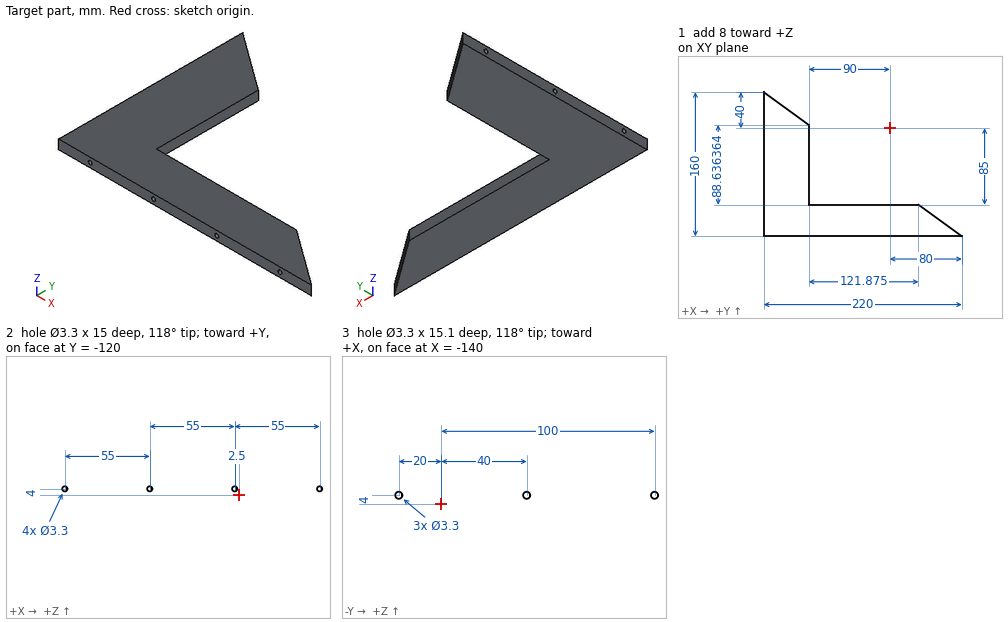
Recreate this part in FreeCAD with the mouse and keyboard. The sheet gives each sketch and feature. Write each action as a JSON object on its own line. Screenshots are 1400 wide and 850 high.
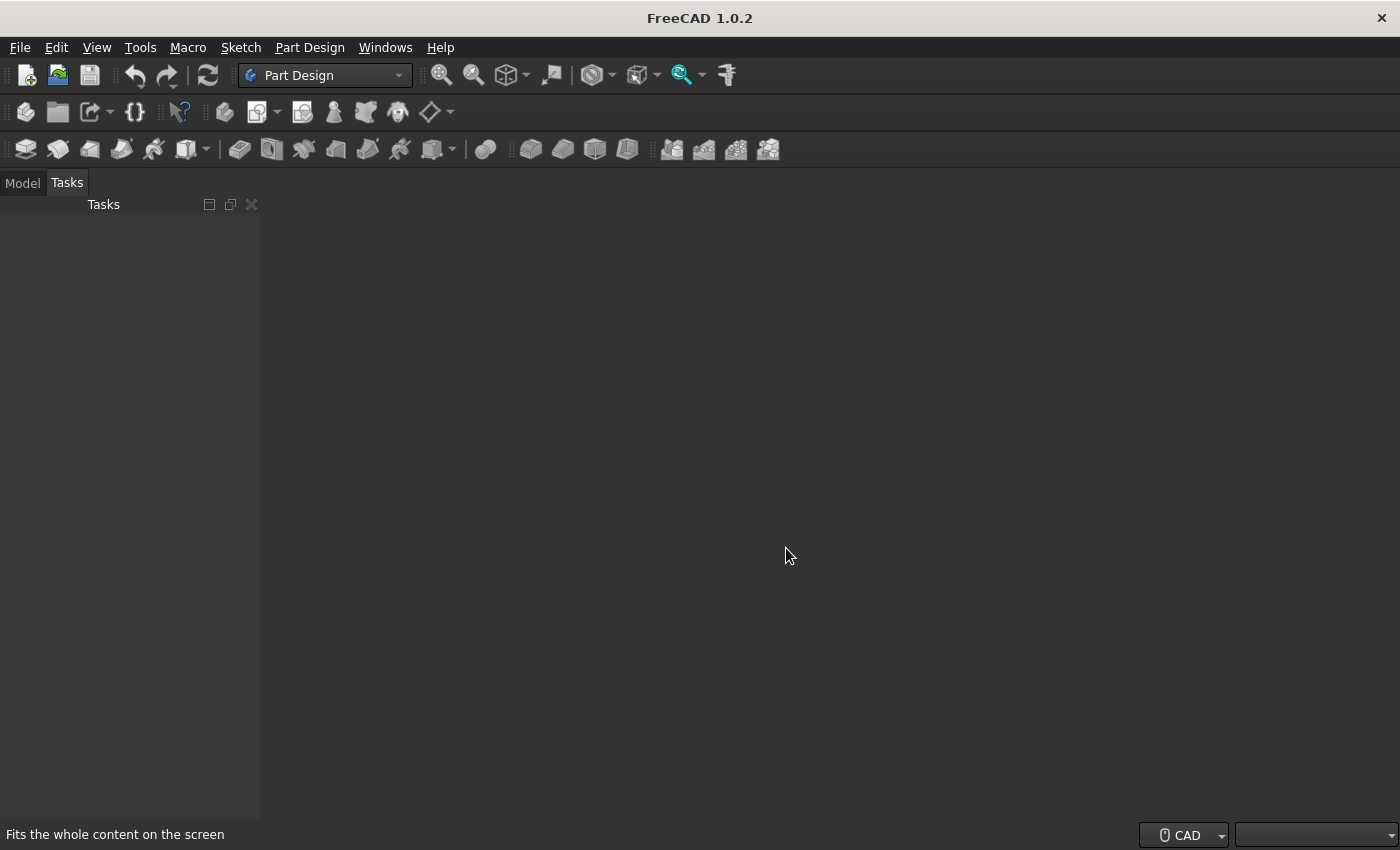
{"action": "key", "text": "ctrl+n"}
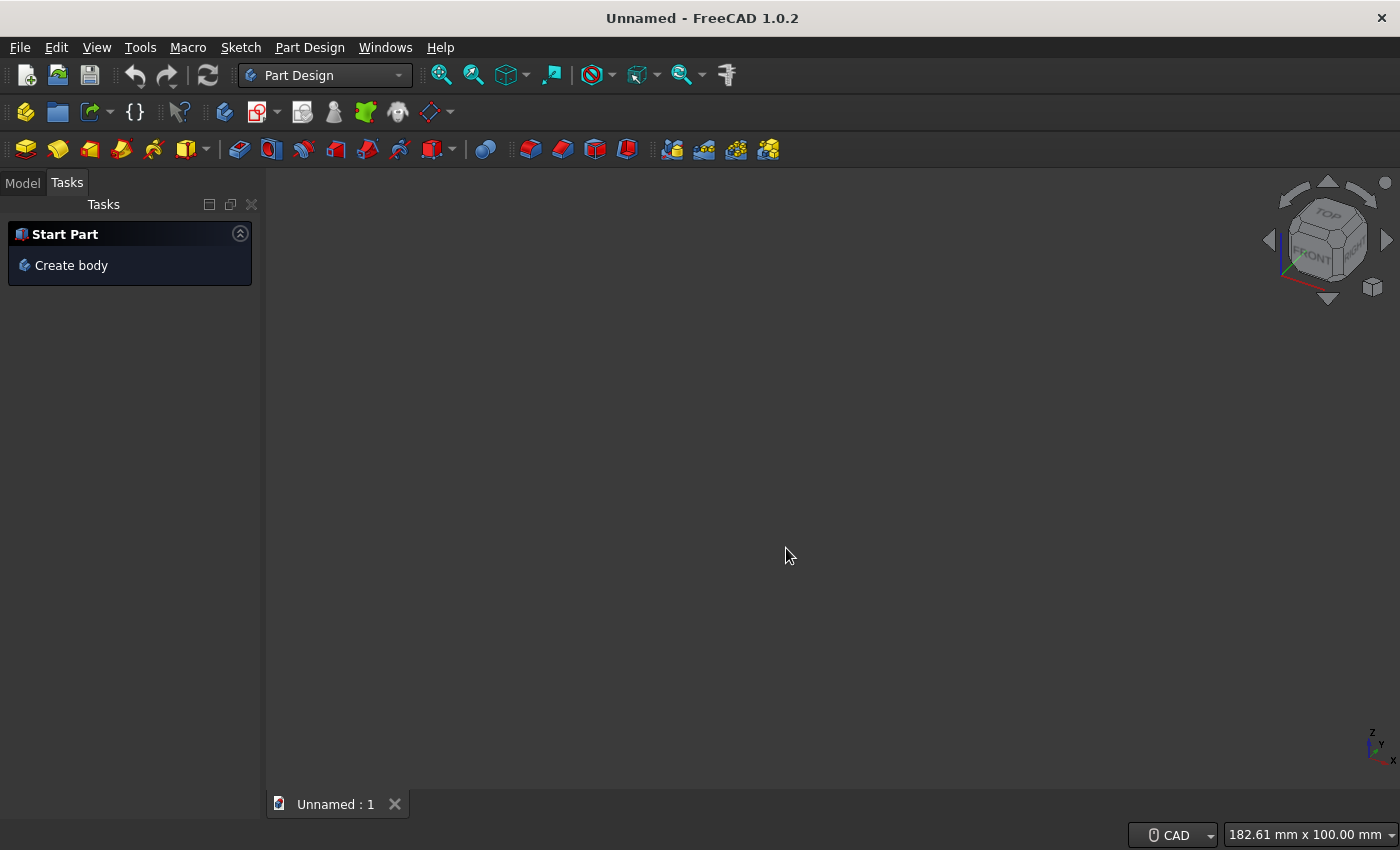
{"action": "left_click", "coordinate": [258, 112]}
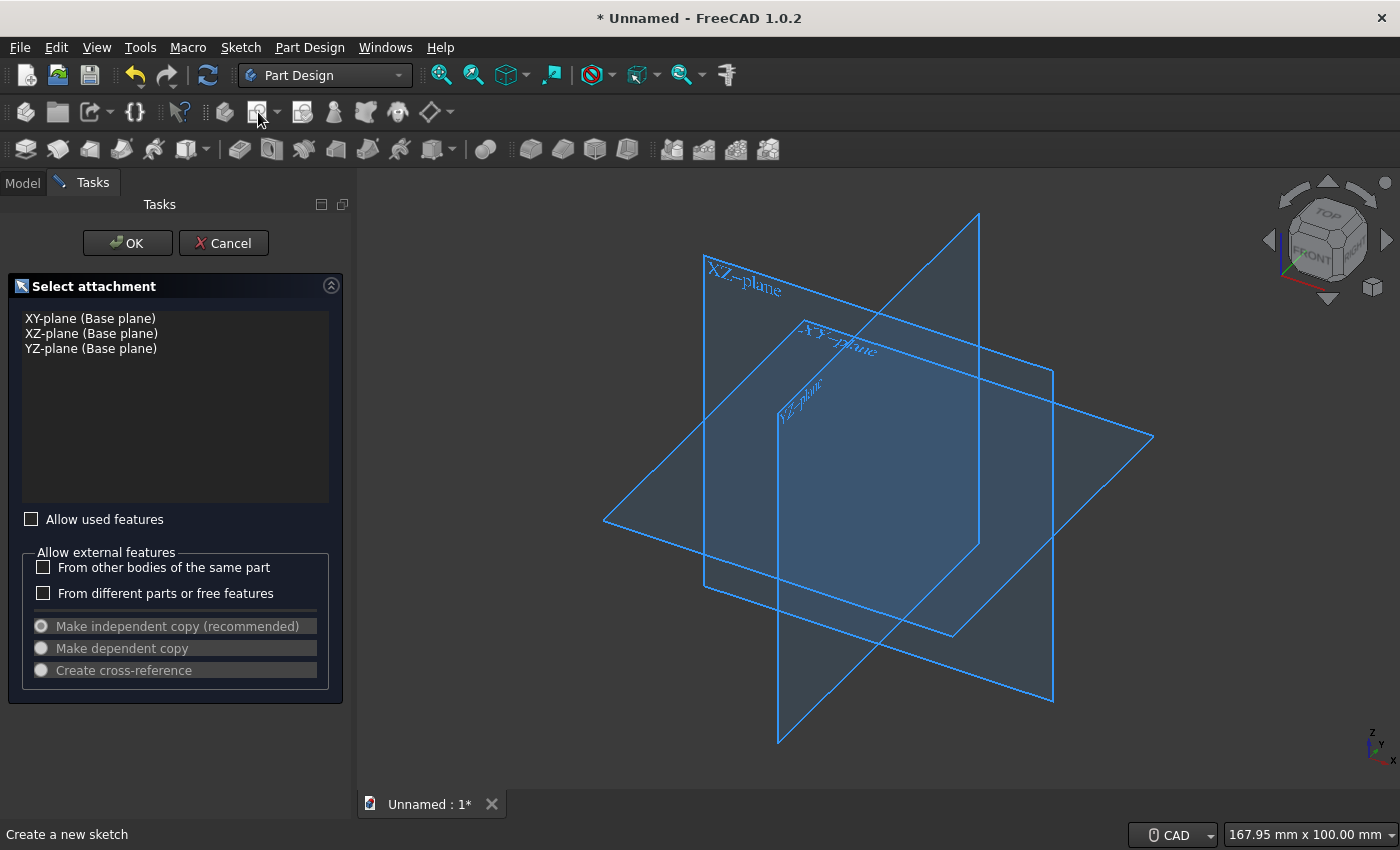
{"action": "left_click", "coordinate": [82, 318]}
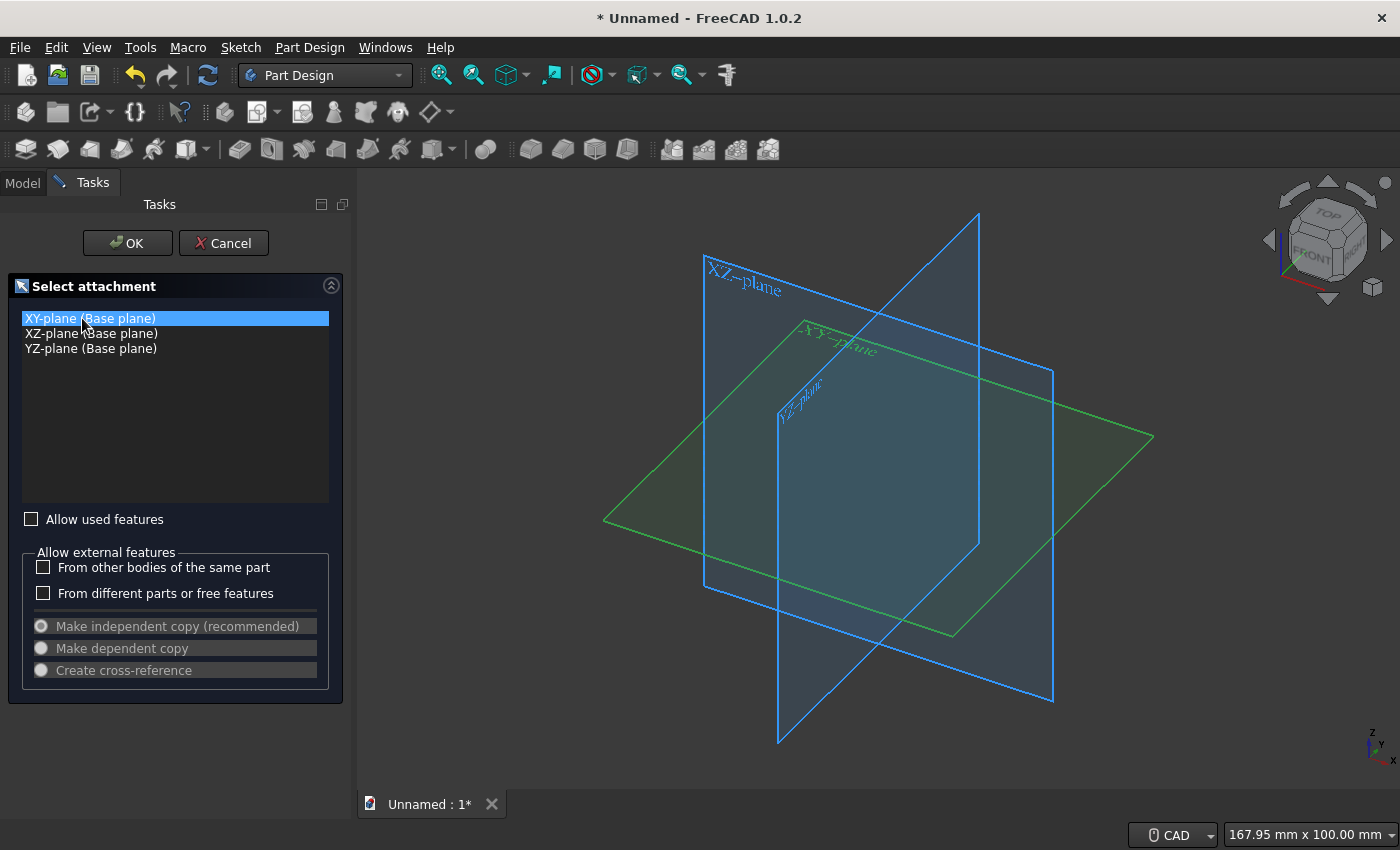
{"action": "left_click", "coordinate": [128, 243]}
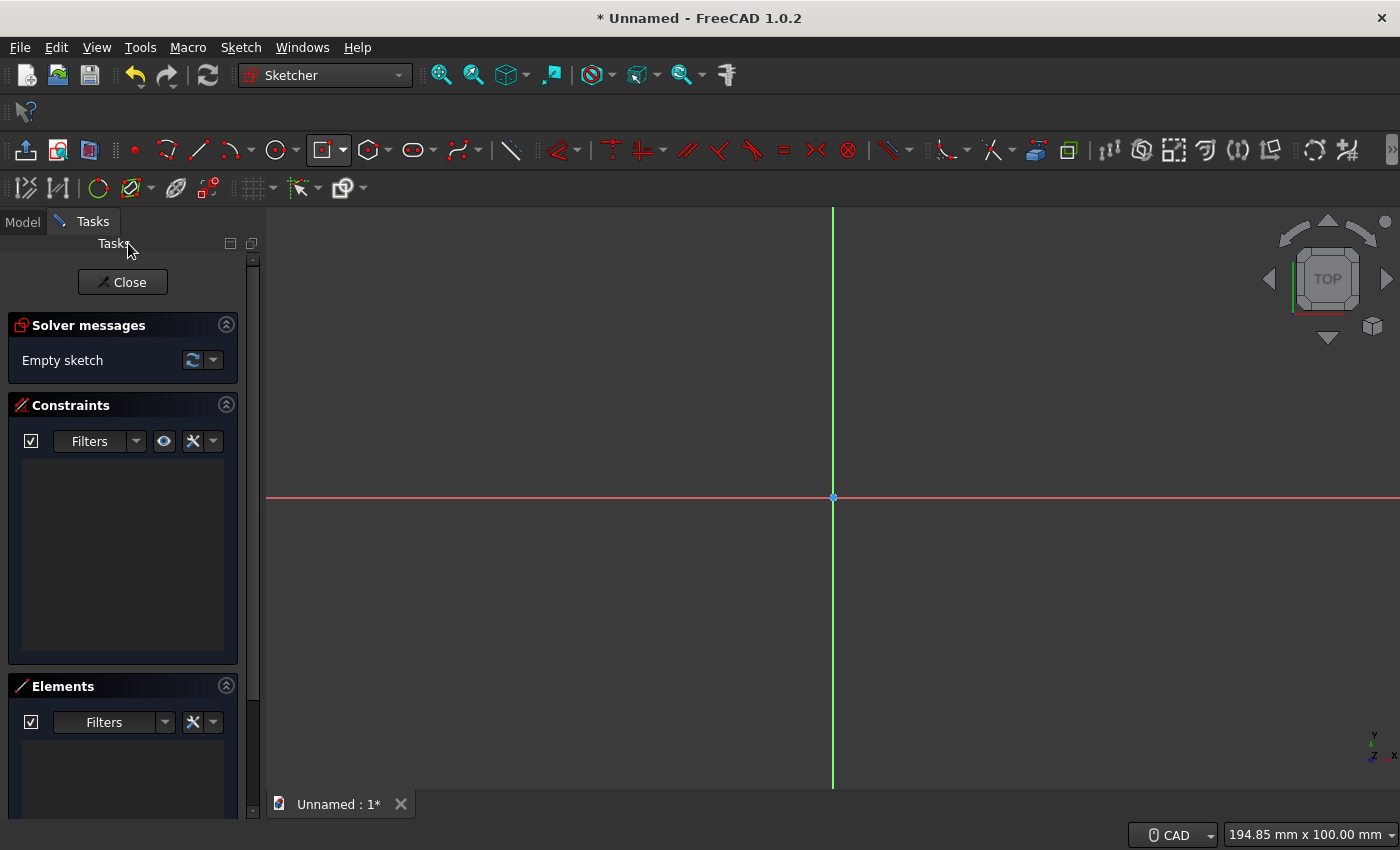
{"action": "scroll", "coordinate": [826, 363], "scroll_direction": "down", "scroll_amount": 5}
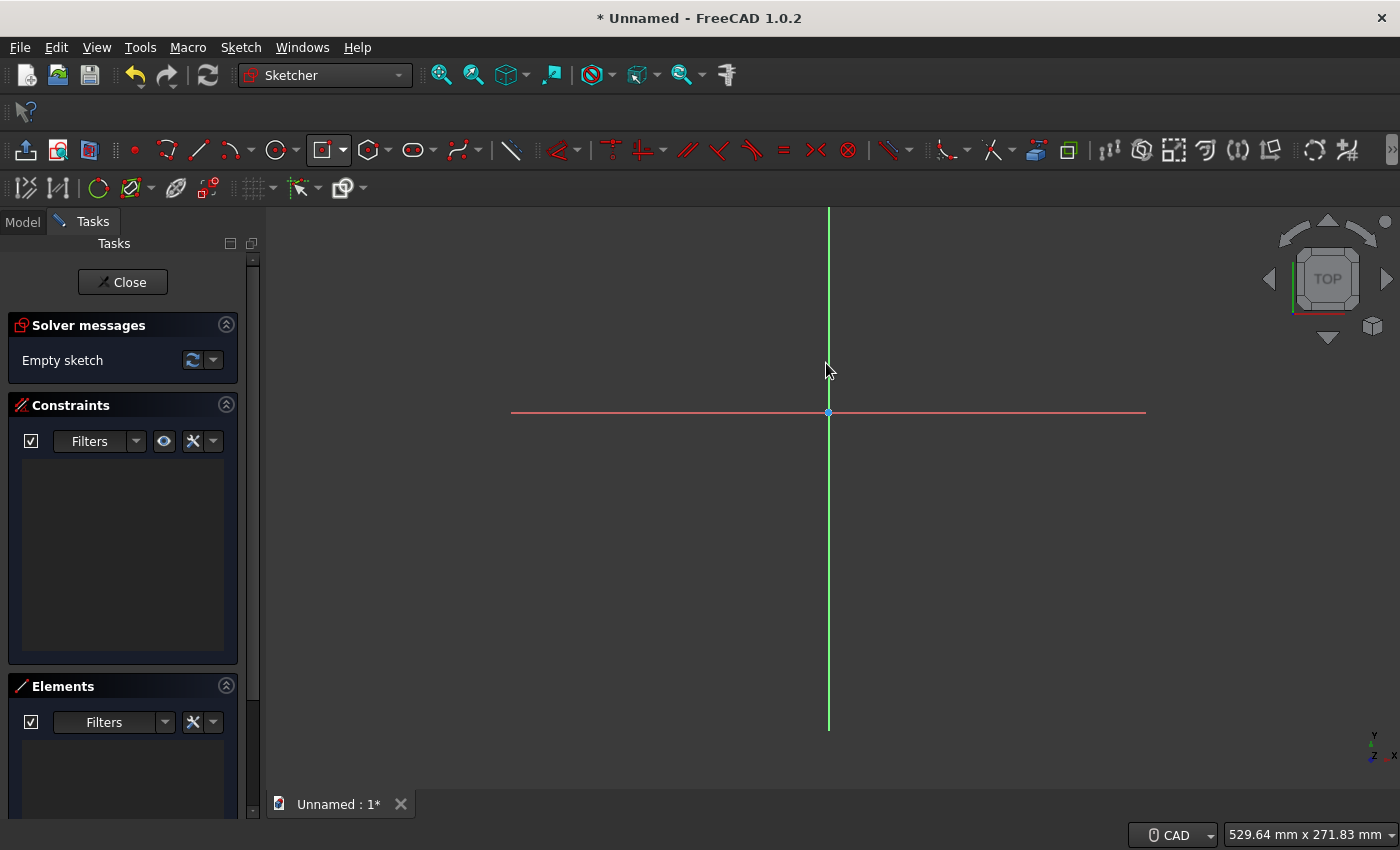
{"action": "key", "text": "g m"}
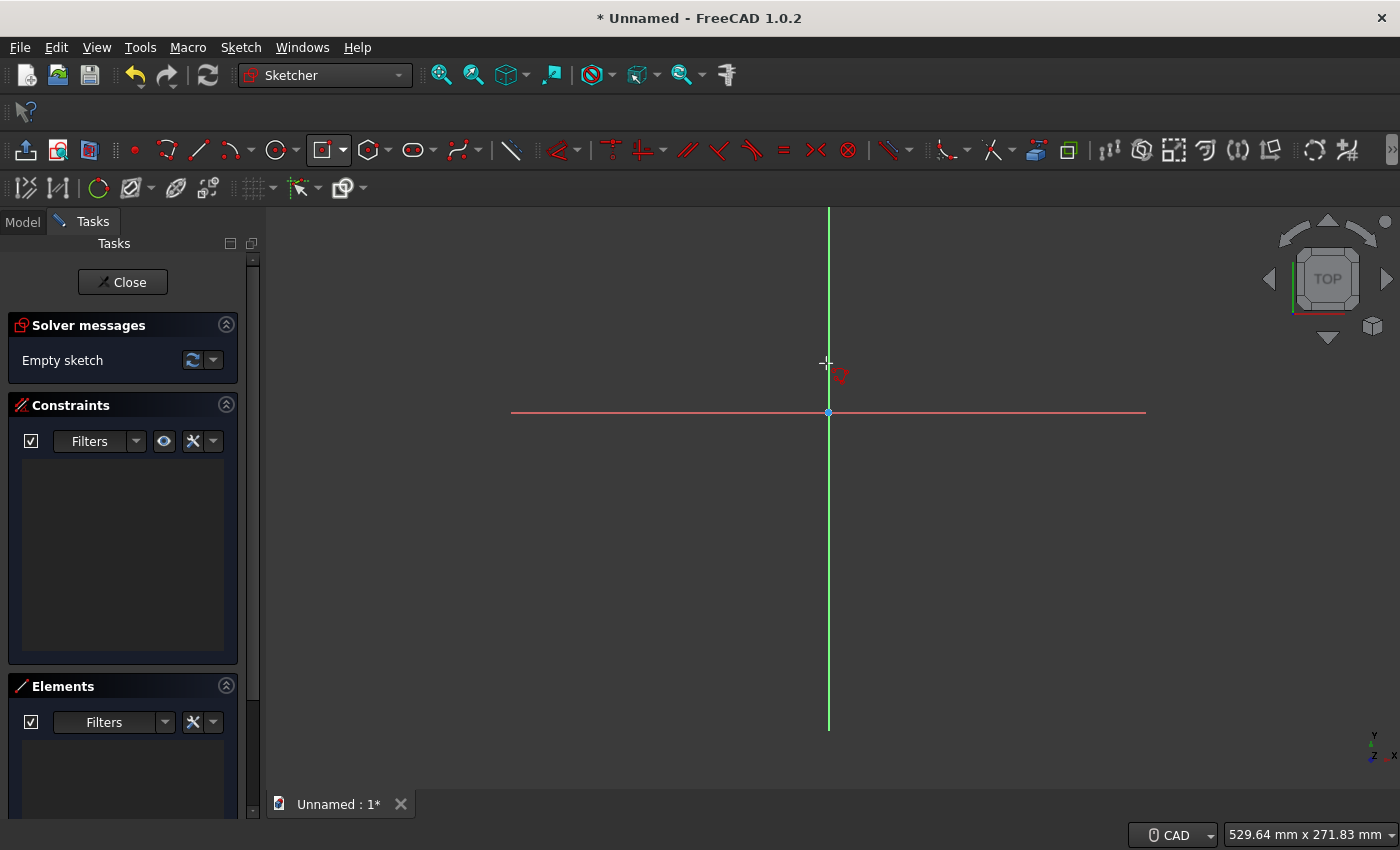
{"action": "scroll", "coordinate": [636, 405], "scroll_direction": "up", "scroll_amount": 4}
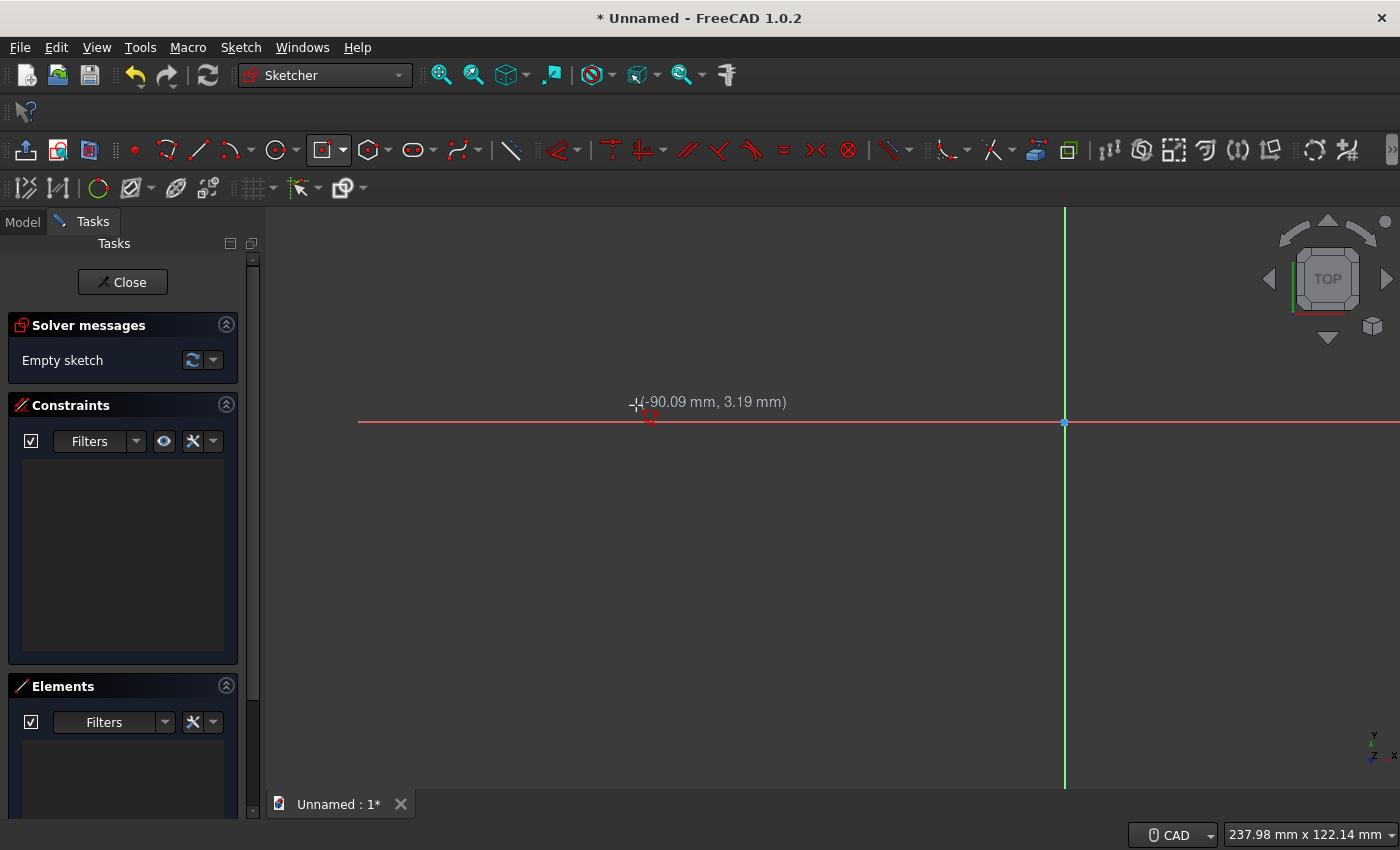
{"action": "left_click", "coordinate": [636, 405]}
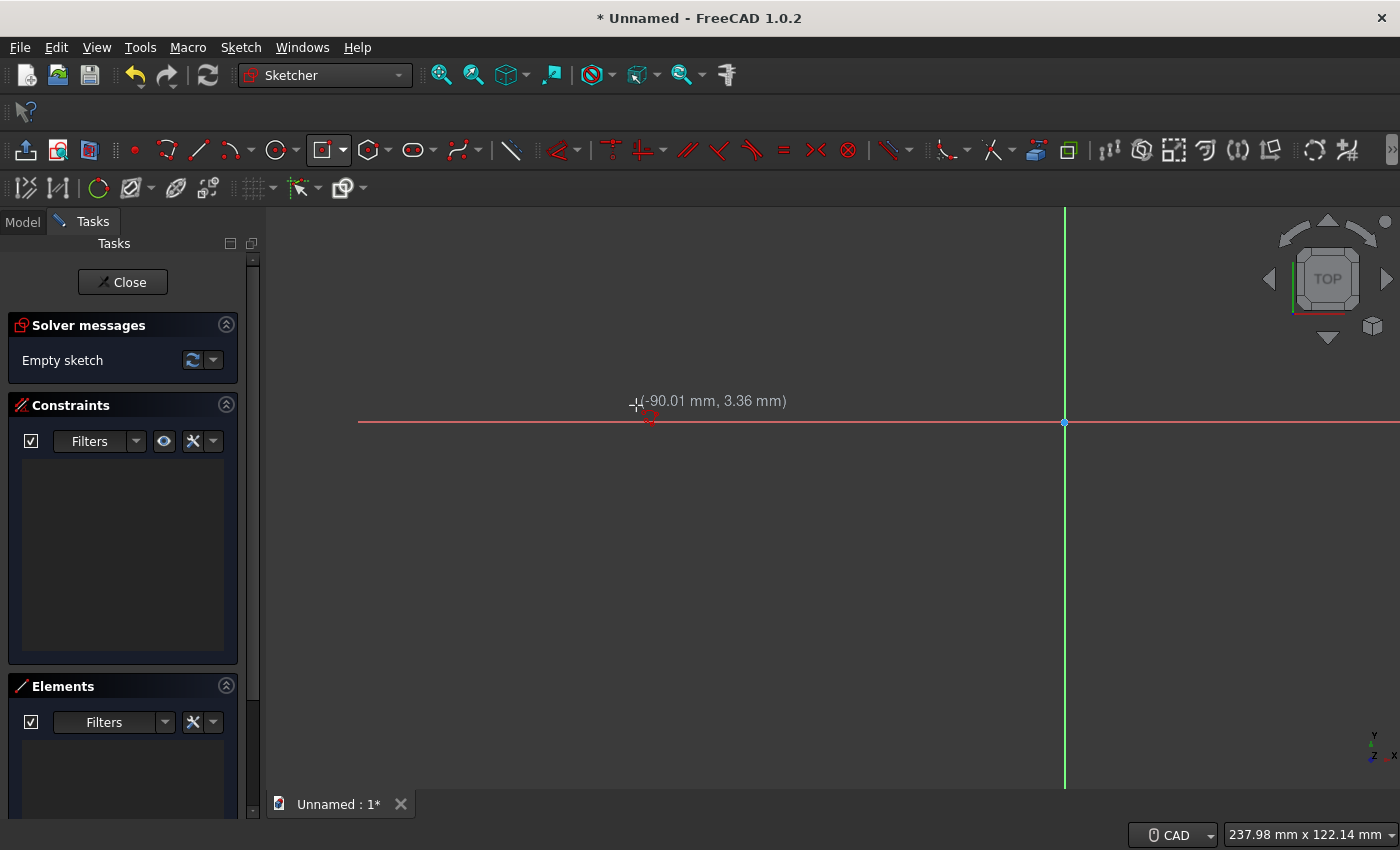
{"action": "scroll", "coordinate": [636, 404], "scroll_direction": "down", "scroll_amount": 4}